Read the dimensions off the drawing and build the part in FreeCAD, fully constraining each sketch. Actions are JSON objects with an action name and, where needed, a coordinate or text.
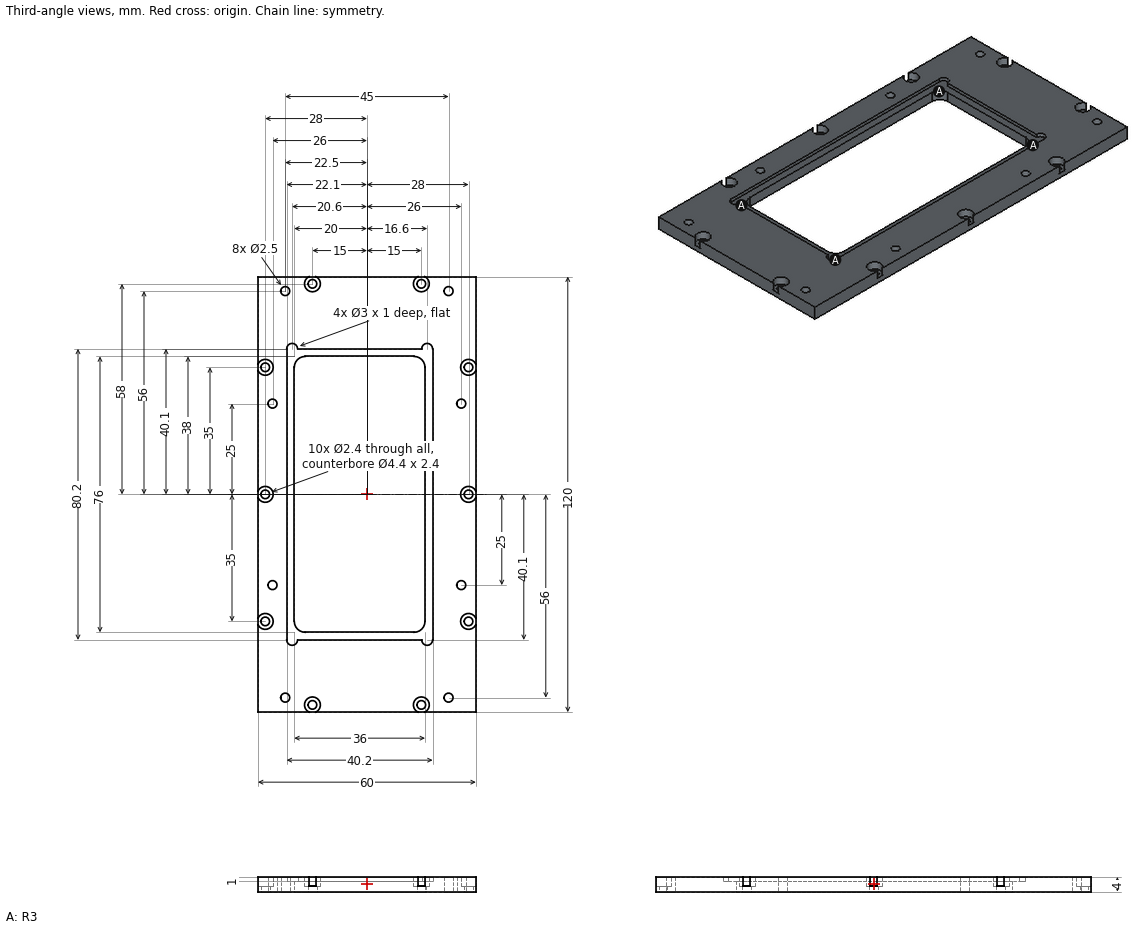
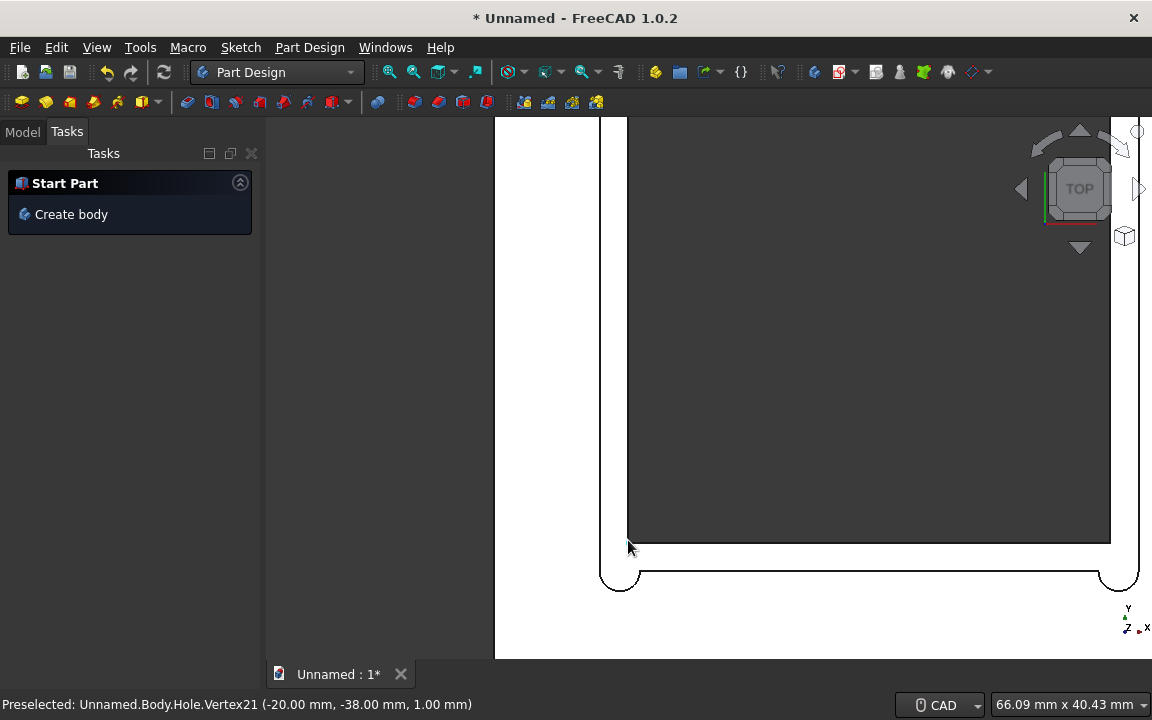
{"action": "key", "text": "v f"}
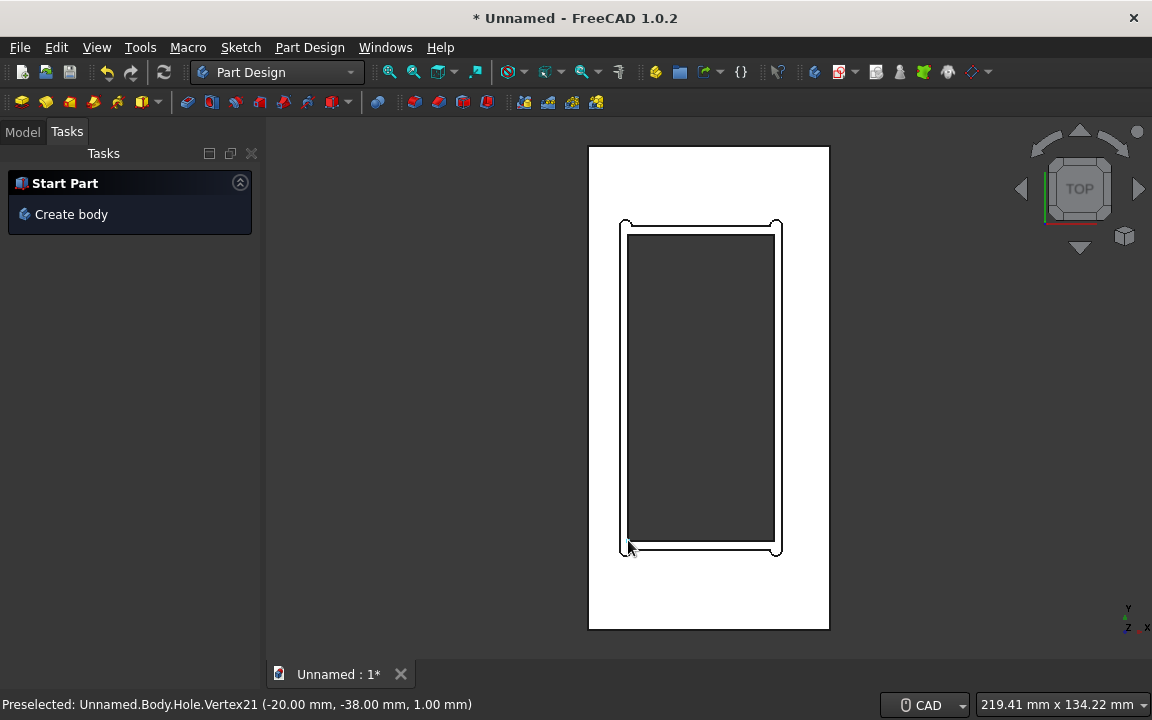
{"action": "key", "text": "1"}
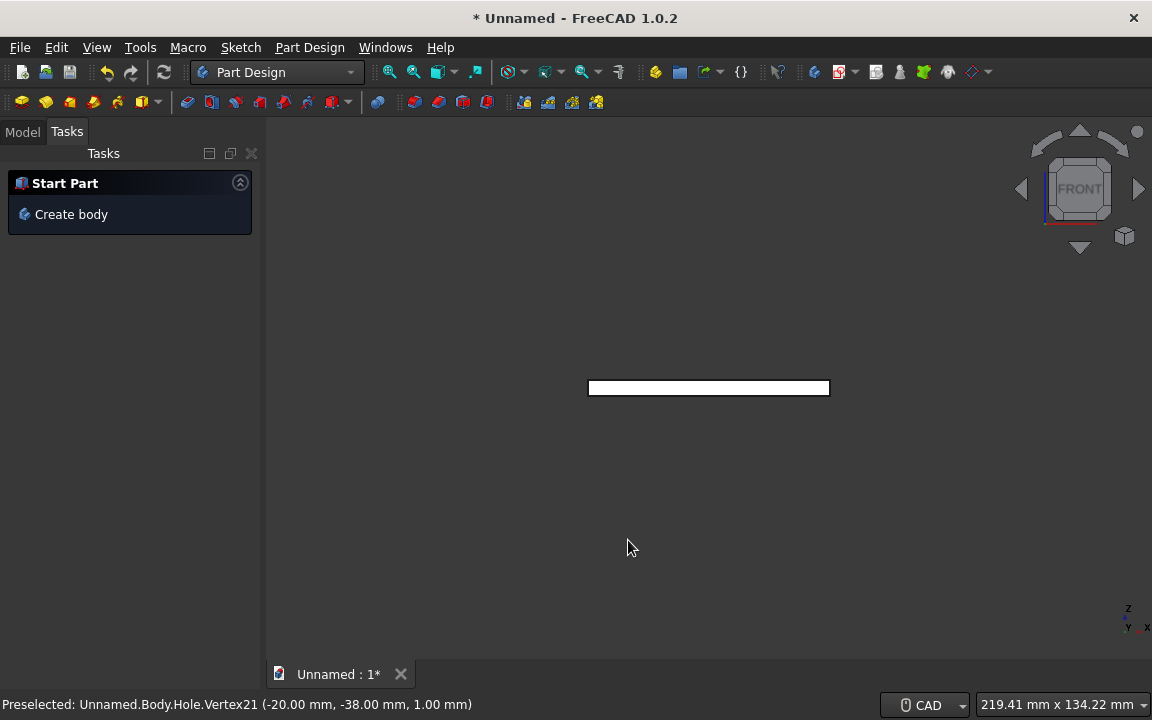
{"action": "left_click", "coordinate": [390, 72]}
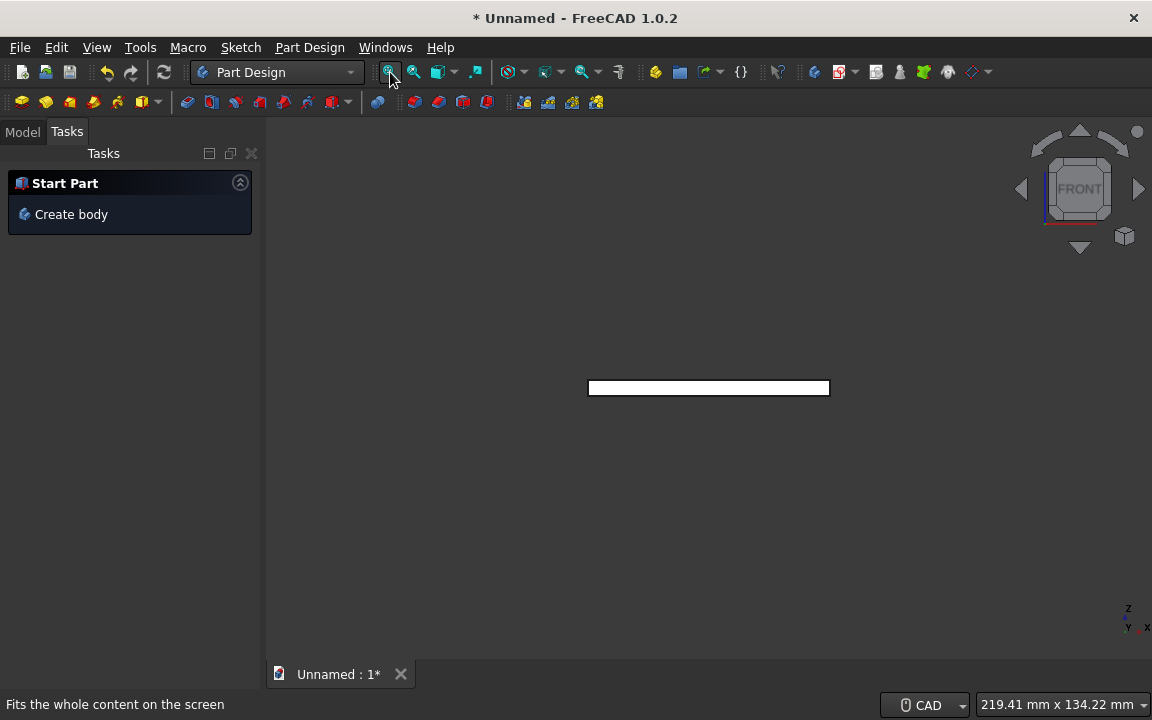
{"action": "scroll", "coordinate": [628, 389], "scroll_direction": "up", "scroll_amount": 6}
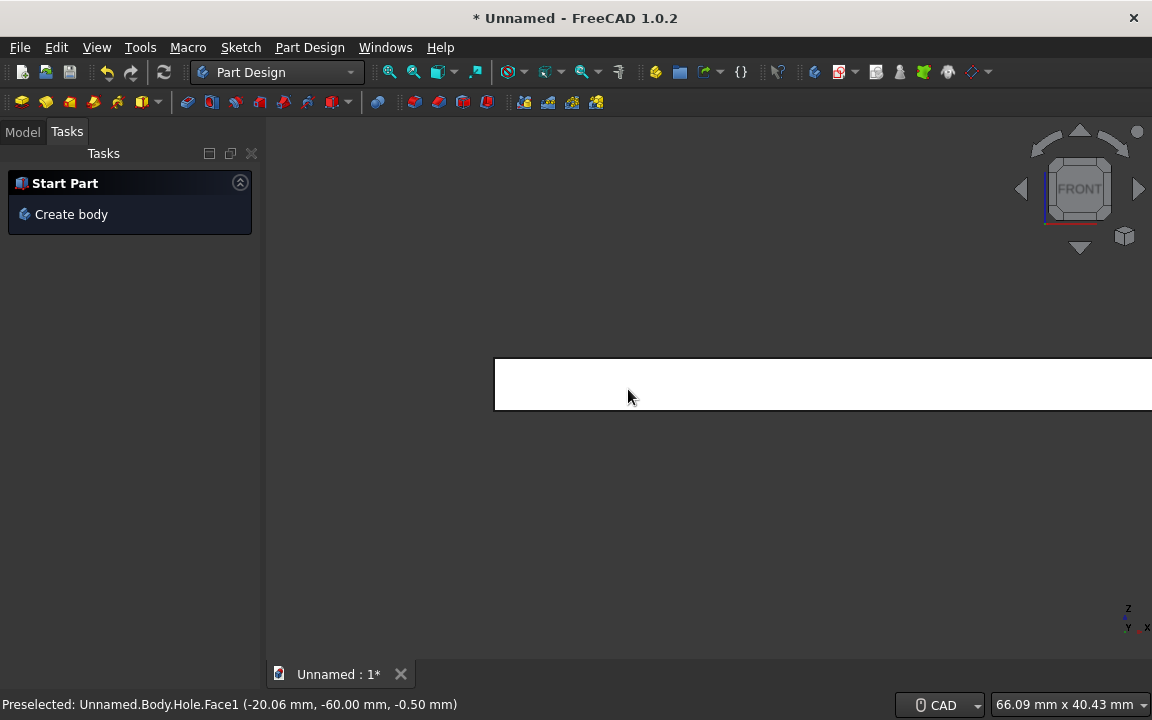
{"action": "key", "text": "v f"}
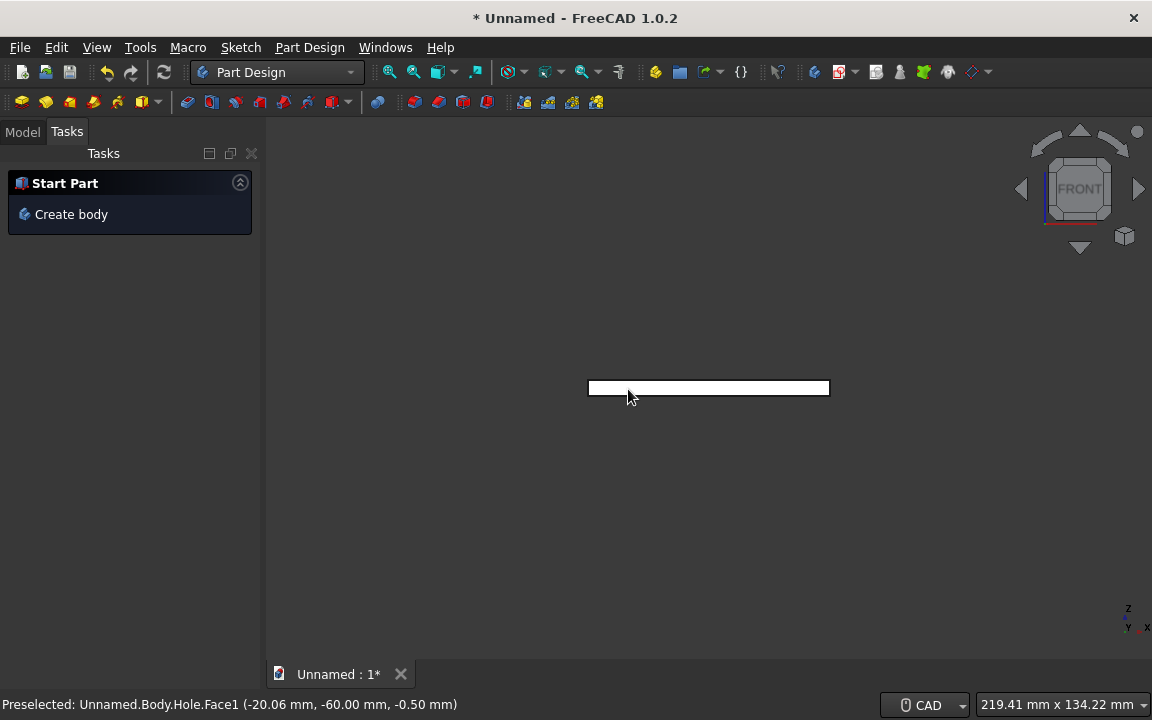
{"action": "key", "text": "3"}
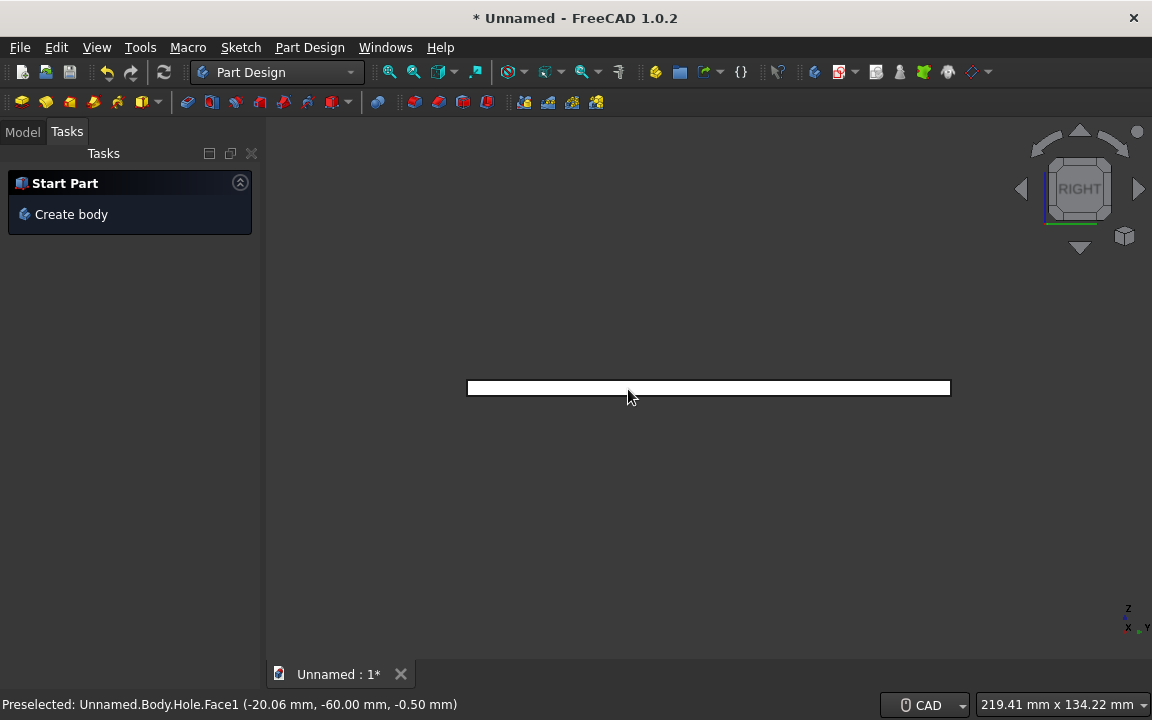
{"action": "scroll", "coordinate": [556, 389], "scroll_direction": "up", "scroll_amount": 6}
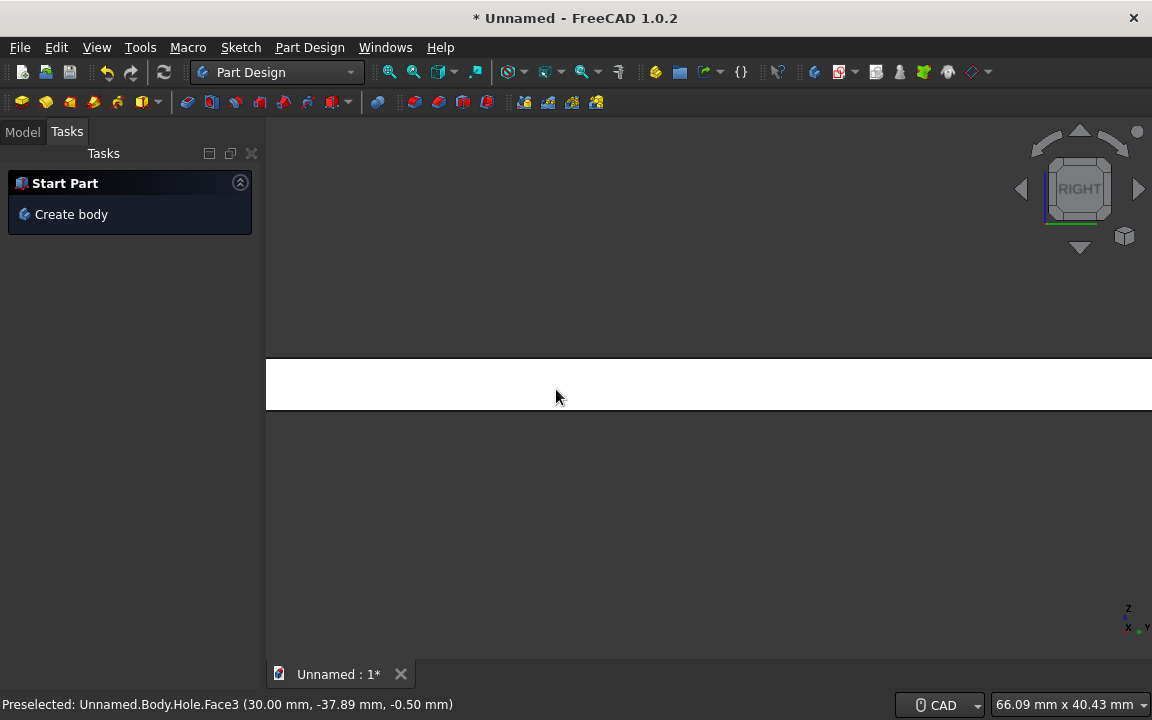
{"action": "key", "text": "v f"}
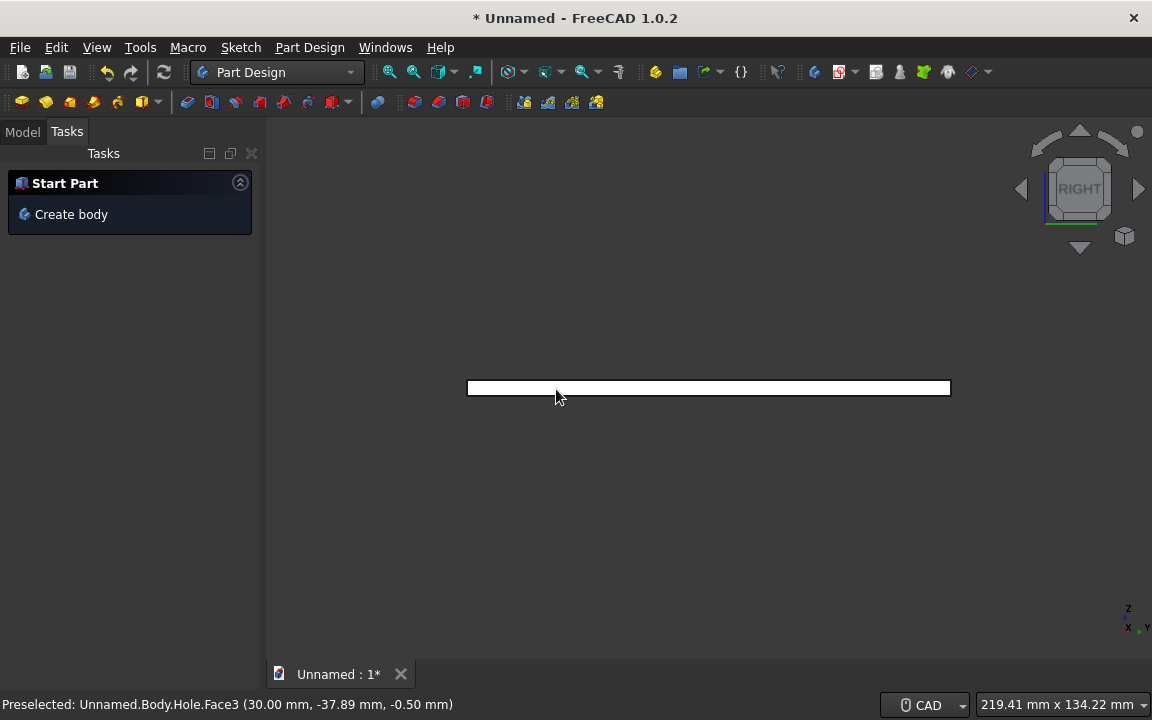
{"action": "key", "text": "5"}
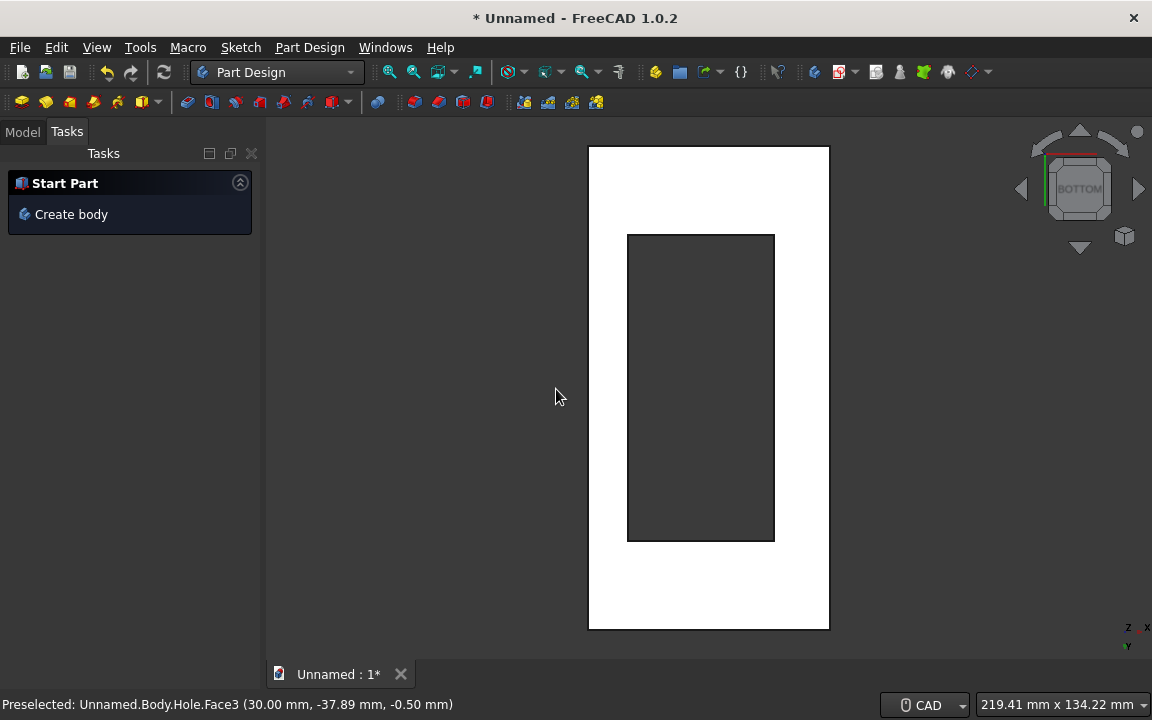
{"action": "scroll", "coordinate": [628, 234], "scroll_direction": "up", "scroll_amount": 6}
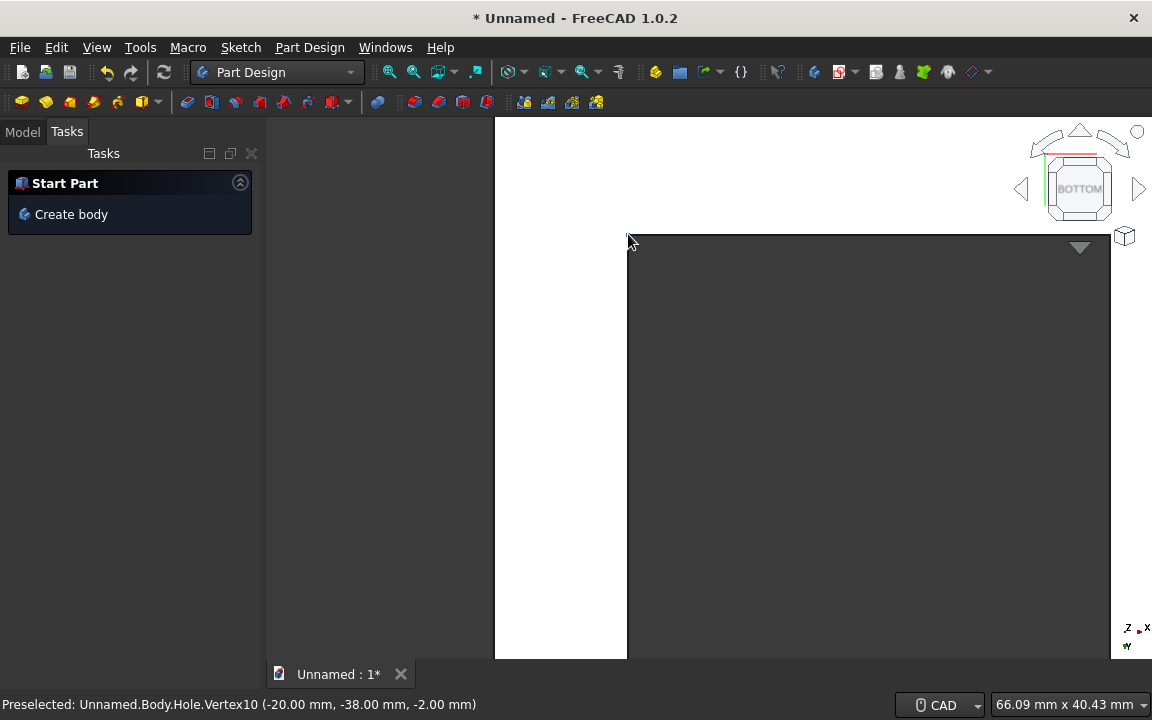
{"action": "key", "text": "v f"}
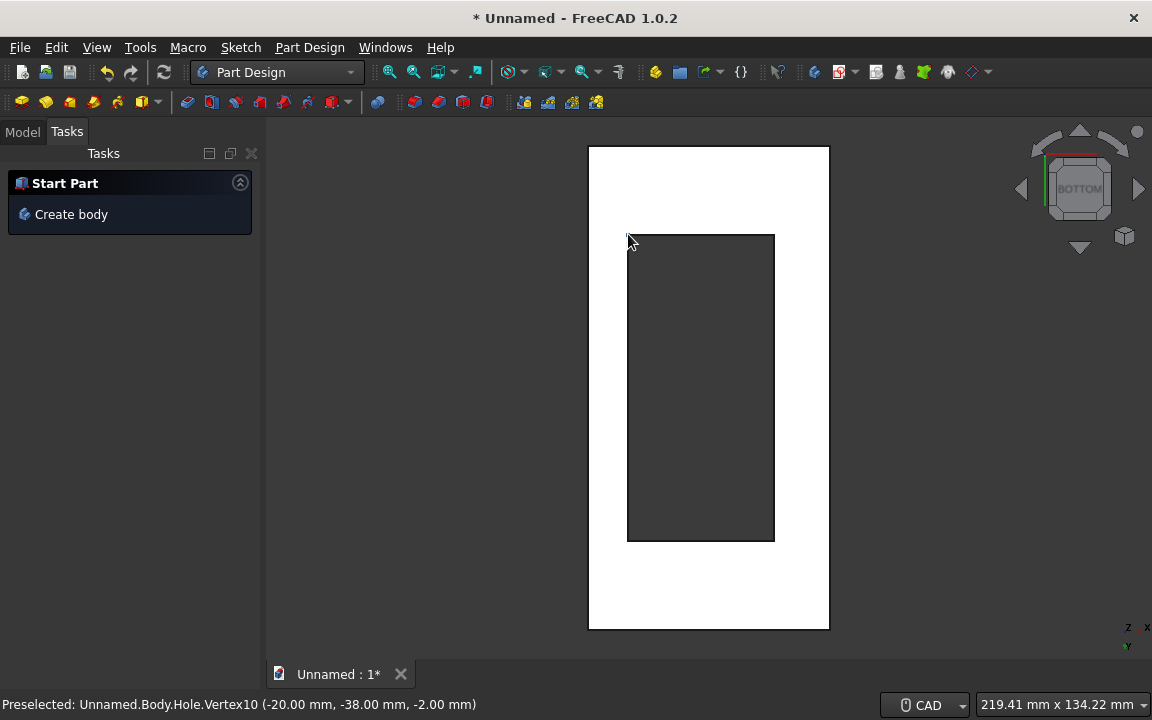
{"action": "key", "text": "4"}